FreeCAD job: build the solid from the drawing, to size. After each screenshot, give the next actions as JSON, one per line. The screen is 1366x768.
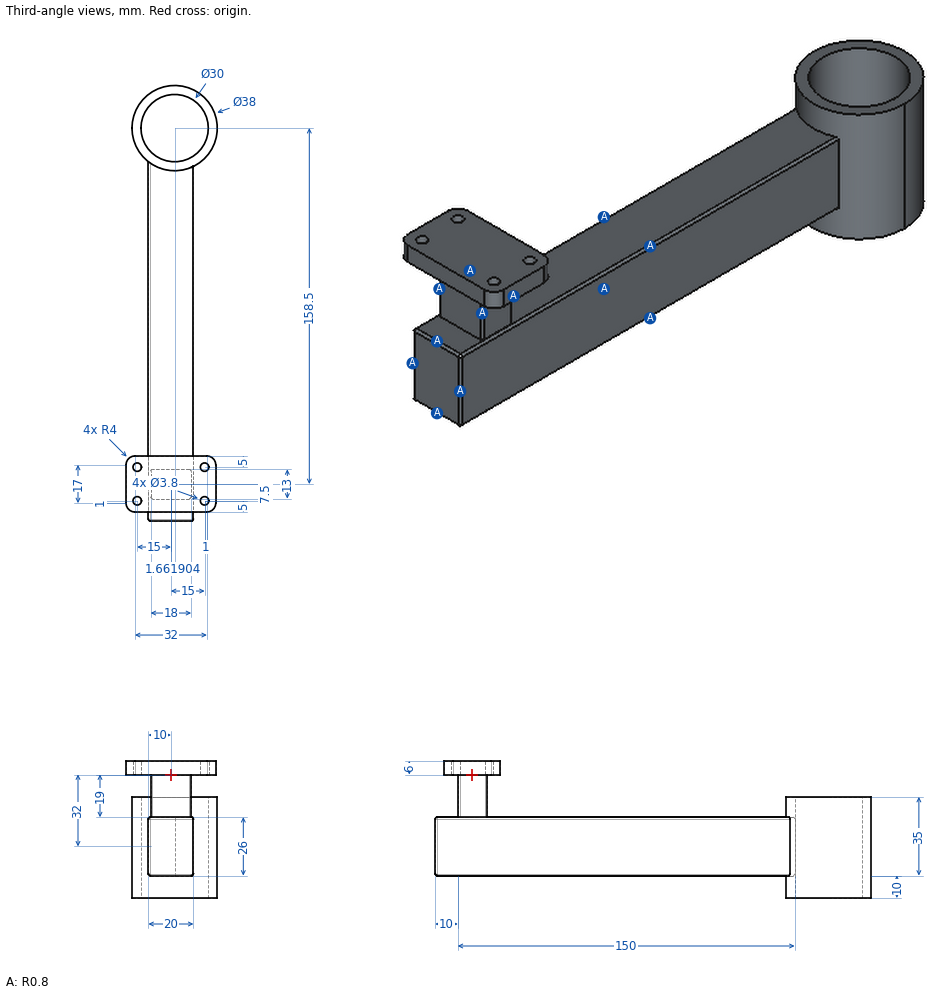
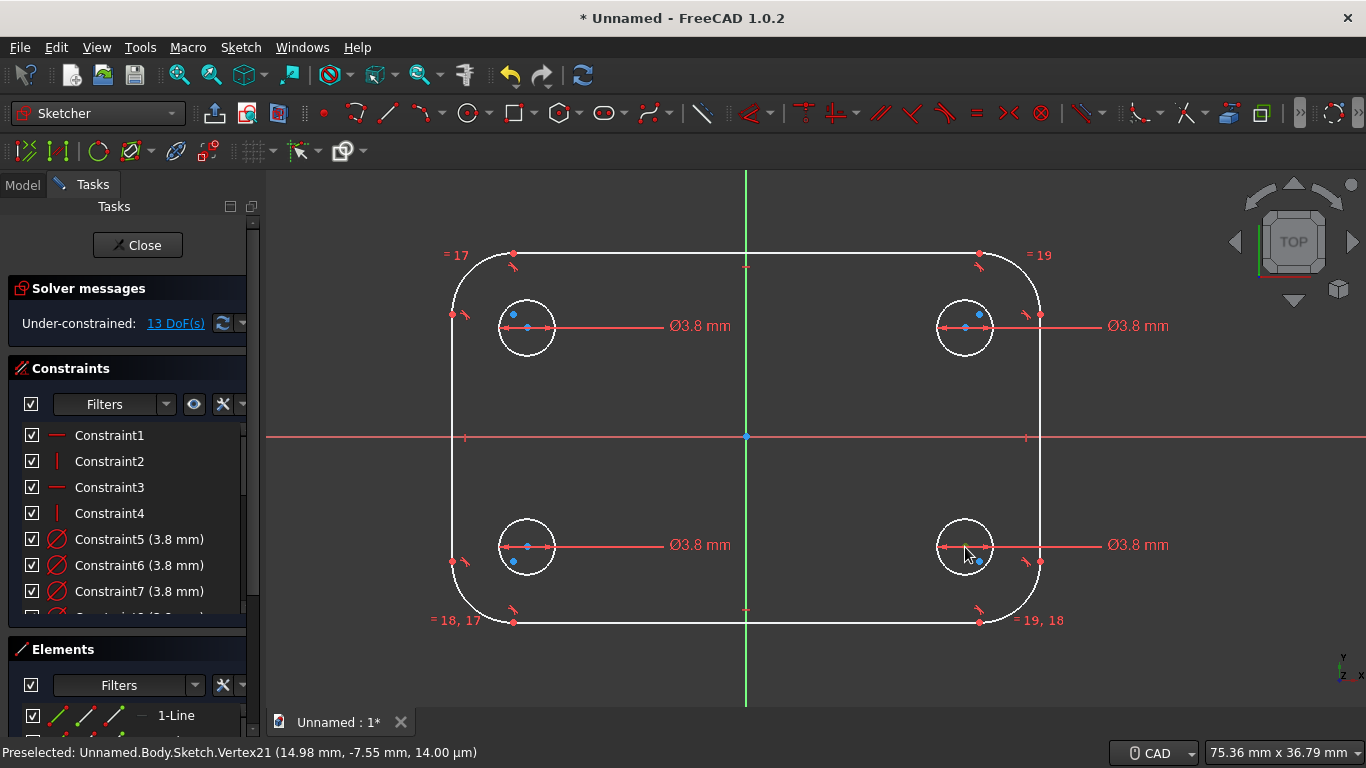
{"action": "left_click", "coordinate": [965, 328]}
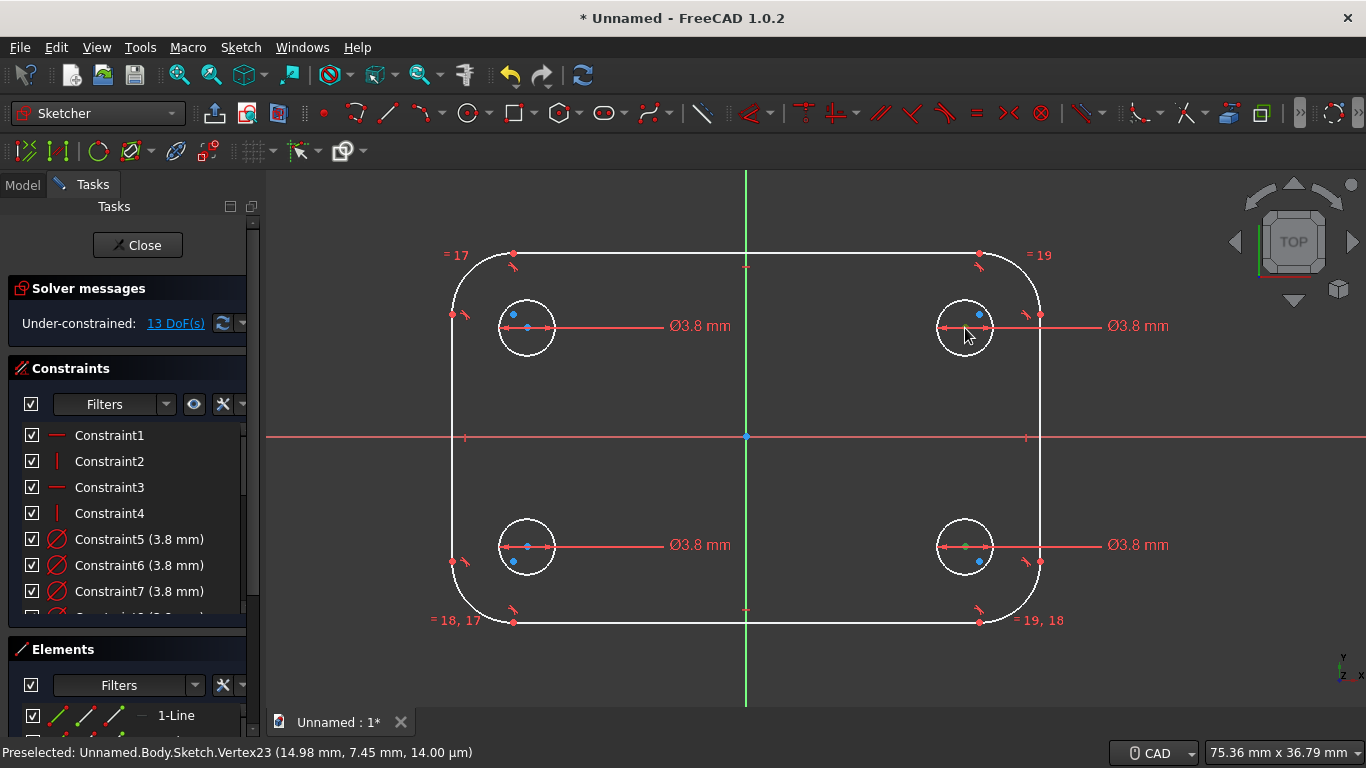
{"action": "left_click", "coordinate": [858, 114]}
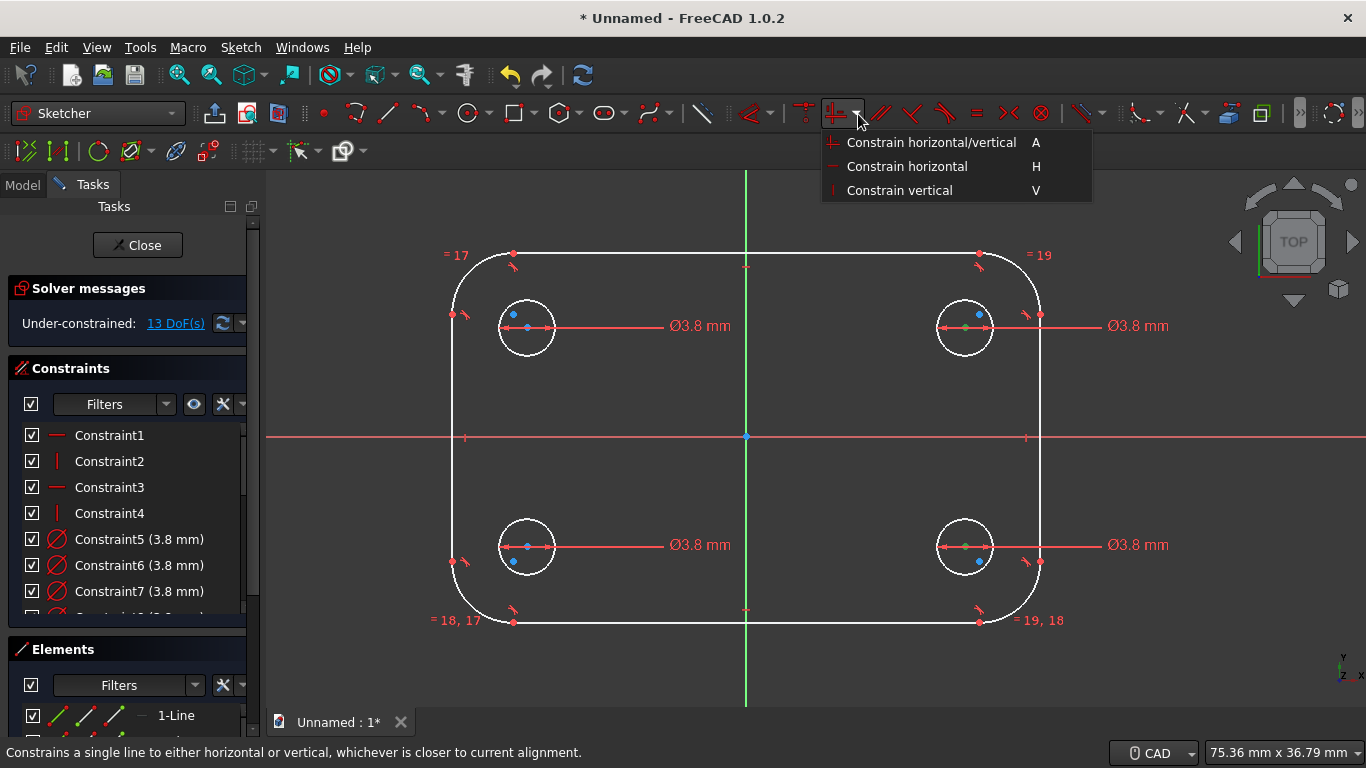
{"action": "left_click", "coordinate": [957, 190]}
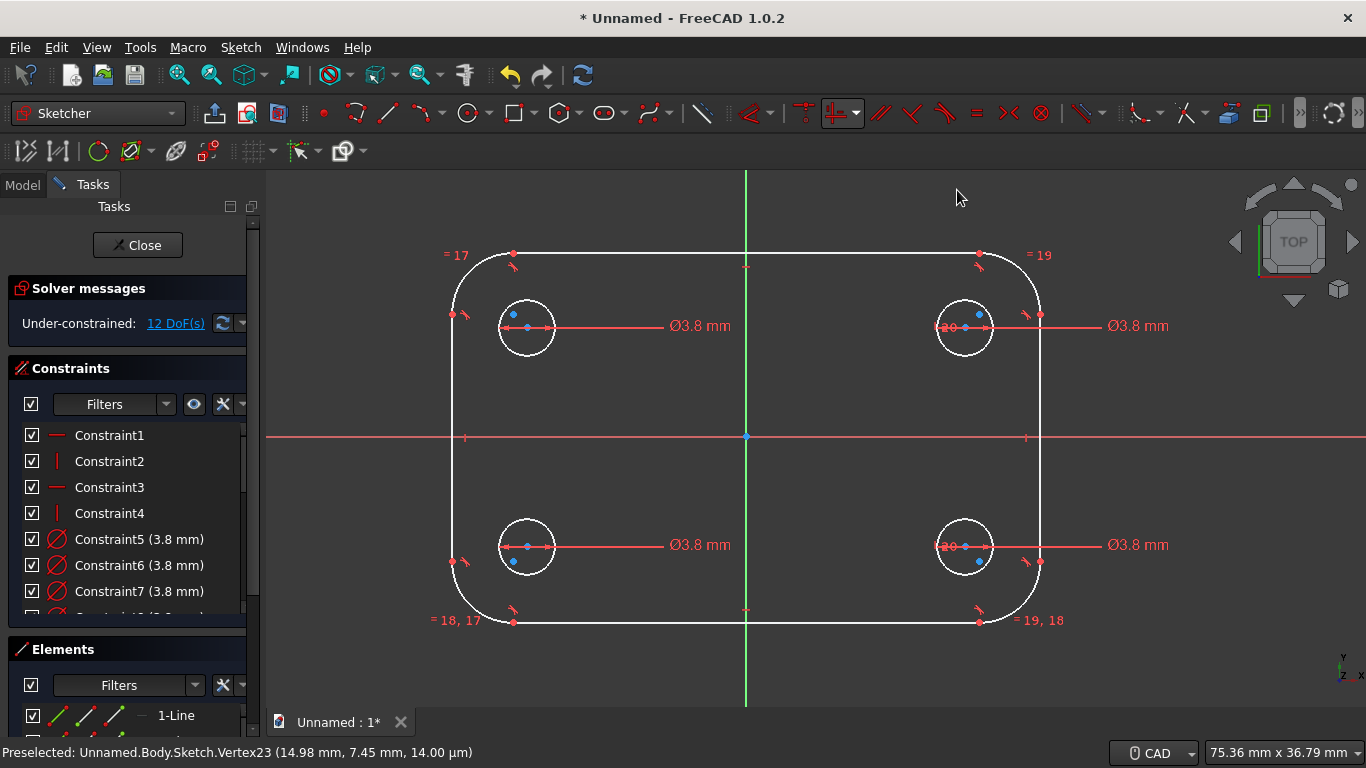
{"action": "left_click", "coordinate": [527, 547]}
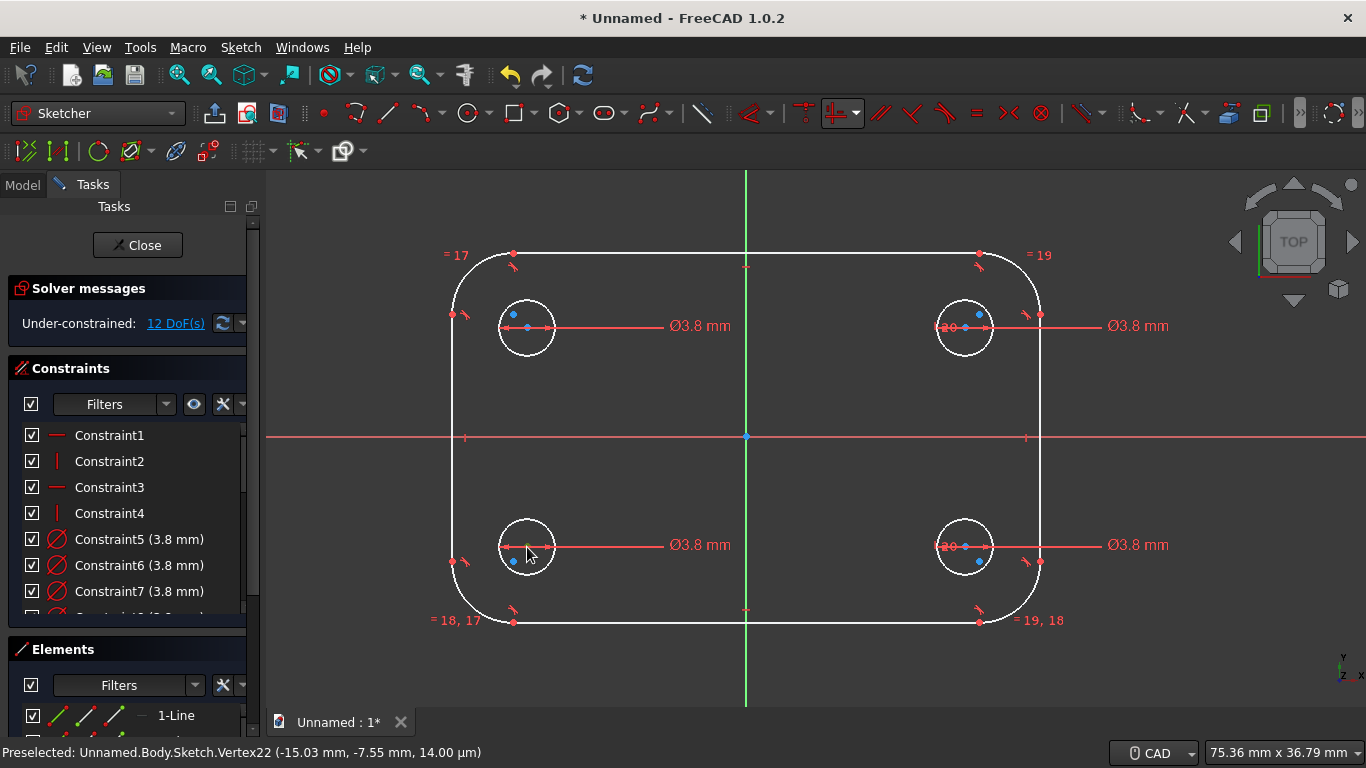
{"action": "left_click", "coordinate": [527, 328]}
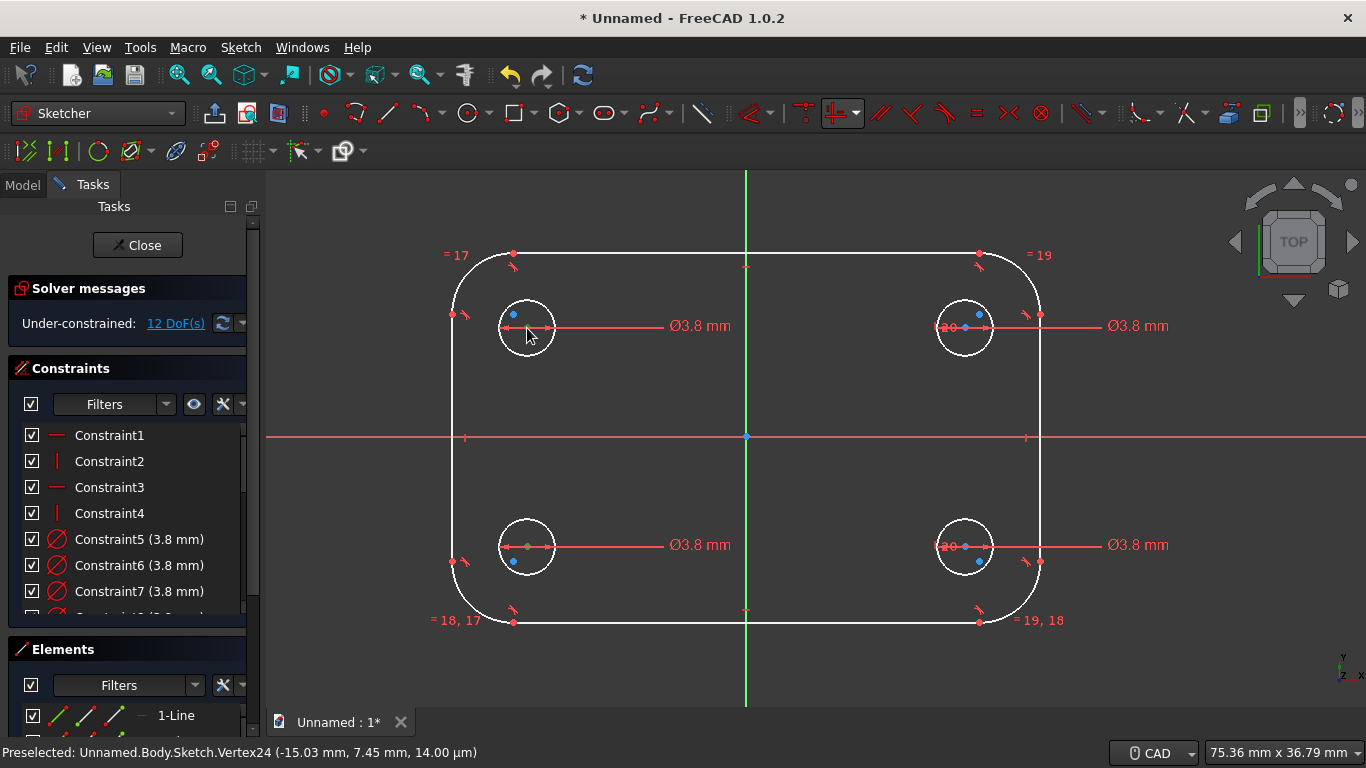
{"action": "left_click", "coordinate": [858, 114]}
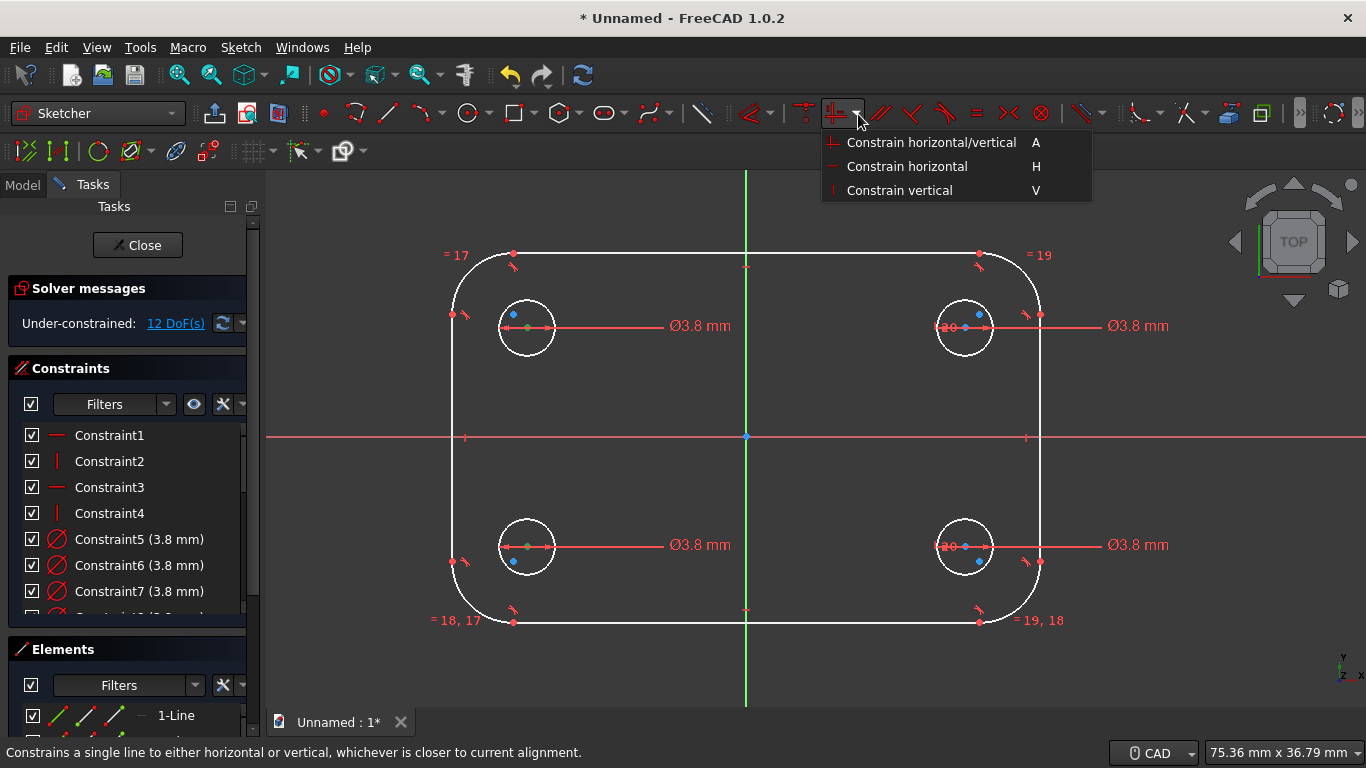
{"action": "left_click", "coordinate": [957, 190]}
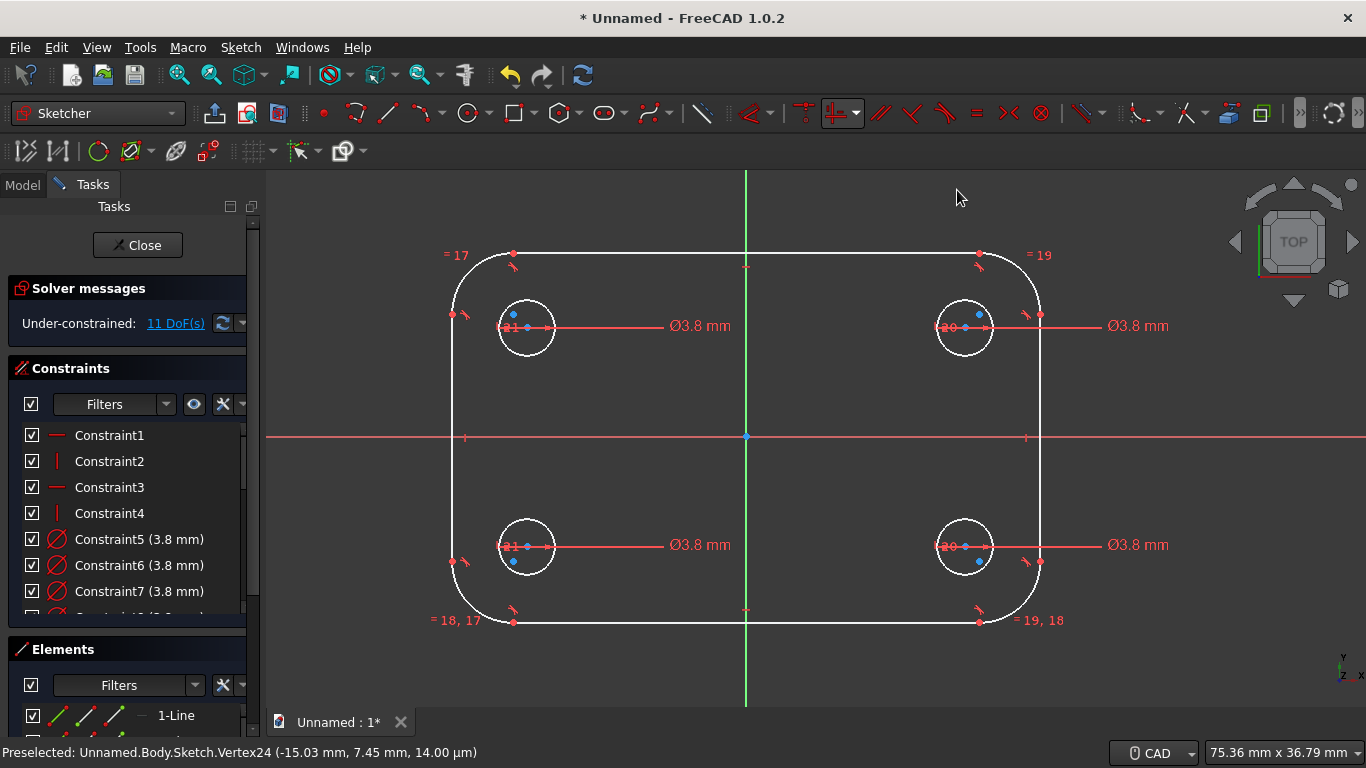
{"action": "left_click", "coordinate": [750, 114]}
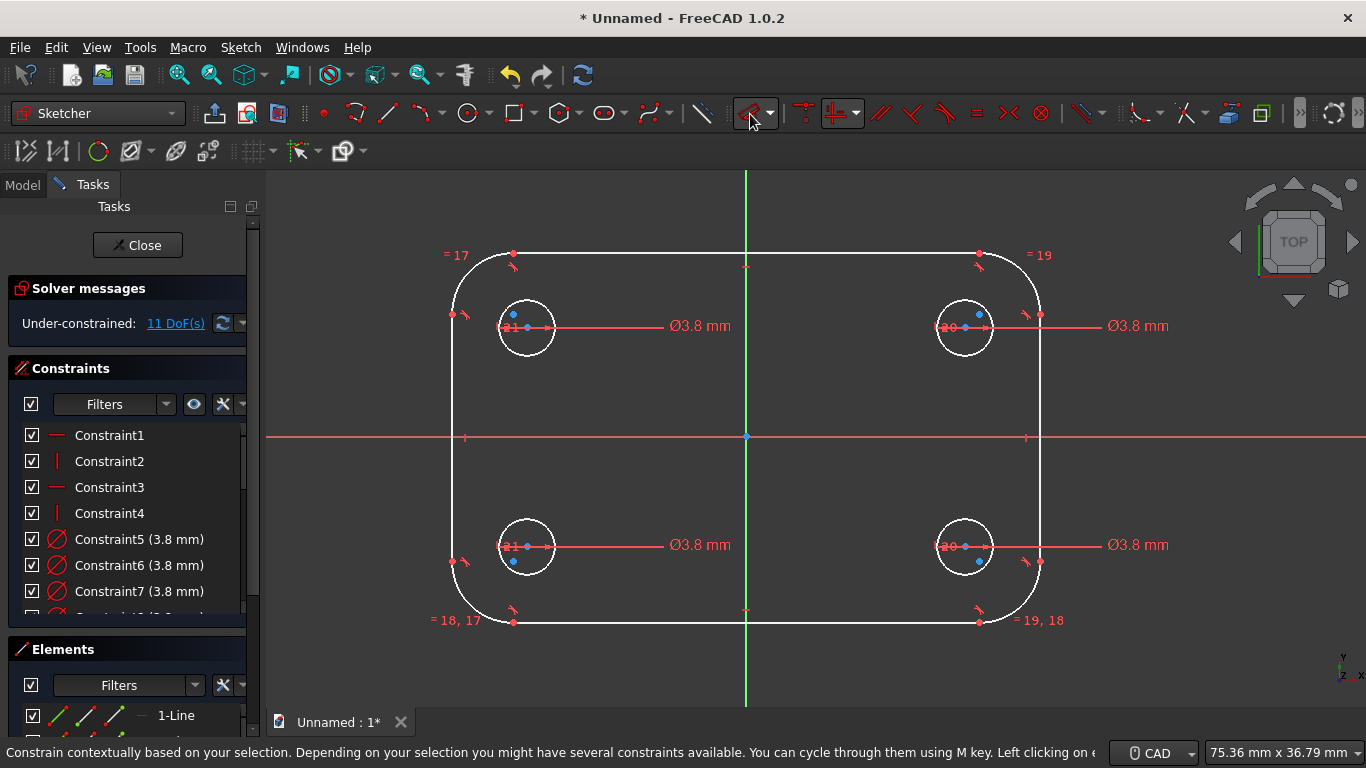
{"action": "left_click", "coordinate": [485, 260]}
{"action": "left_click", "coordinate": [470, 232]}